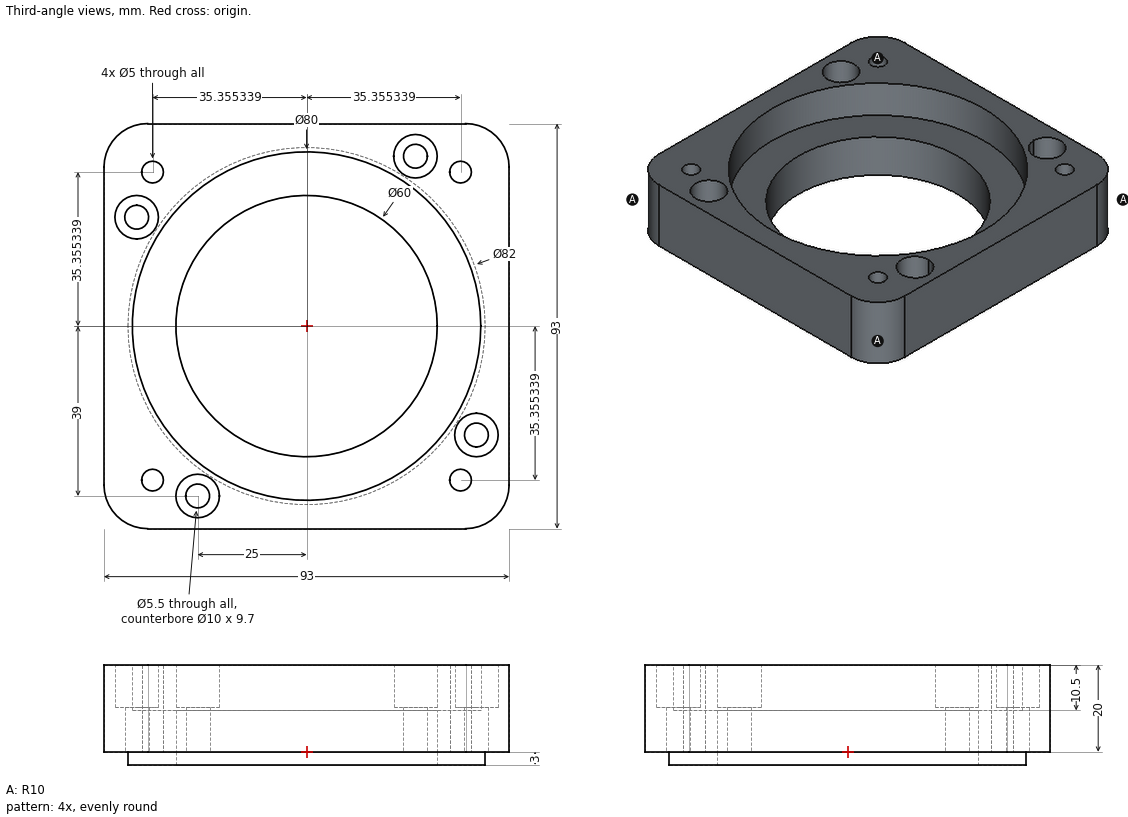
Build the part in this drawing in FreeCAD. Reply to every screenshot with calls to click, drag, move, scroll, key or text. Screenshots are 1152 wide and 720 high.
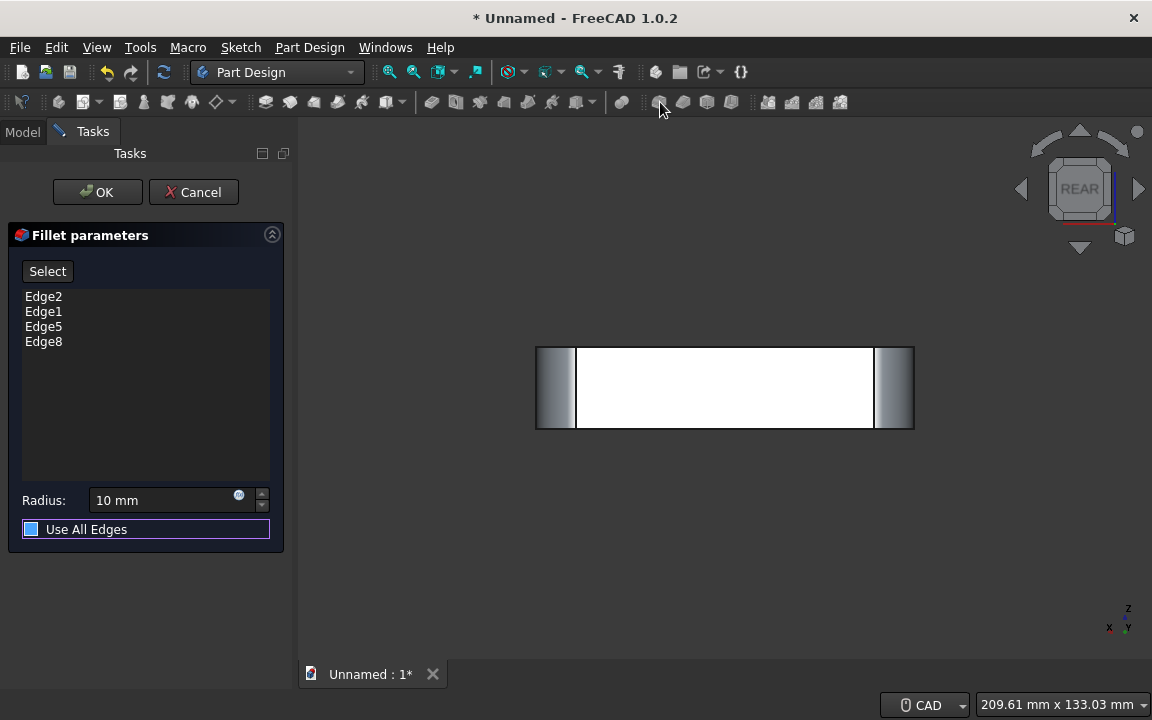
click(98, 192)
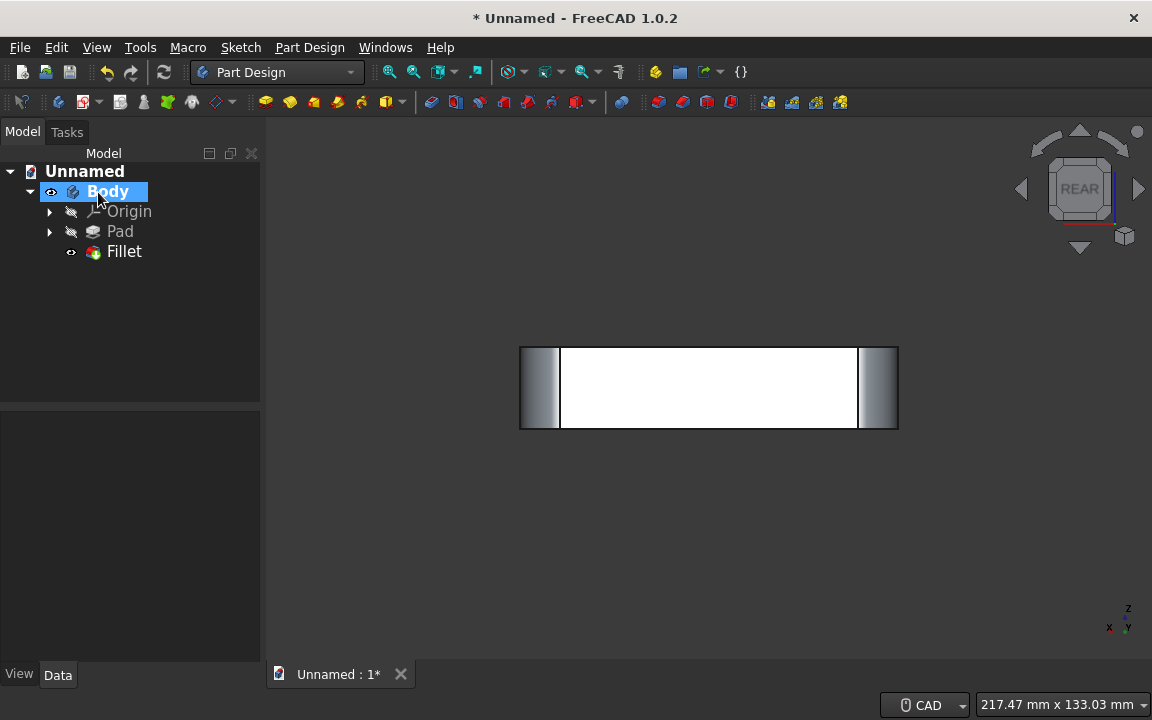
click(390, 72)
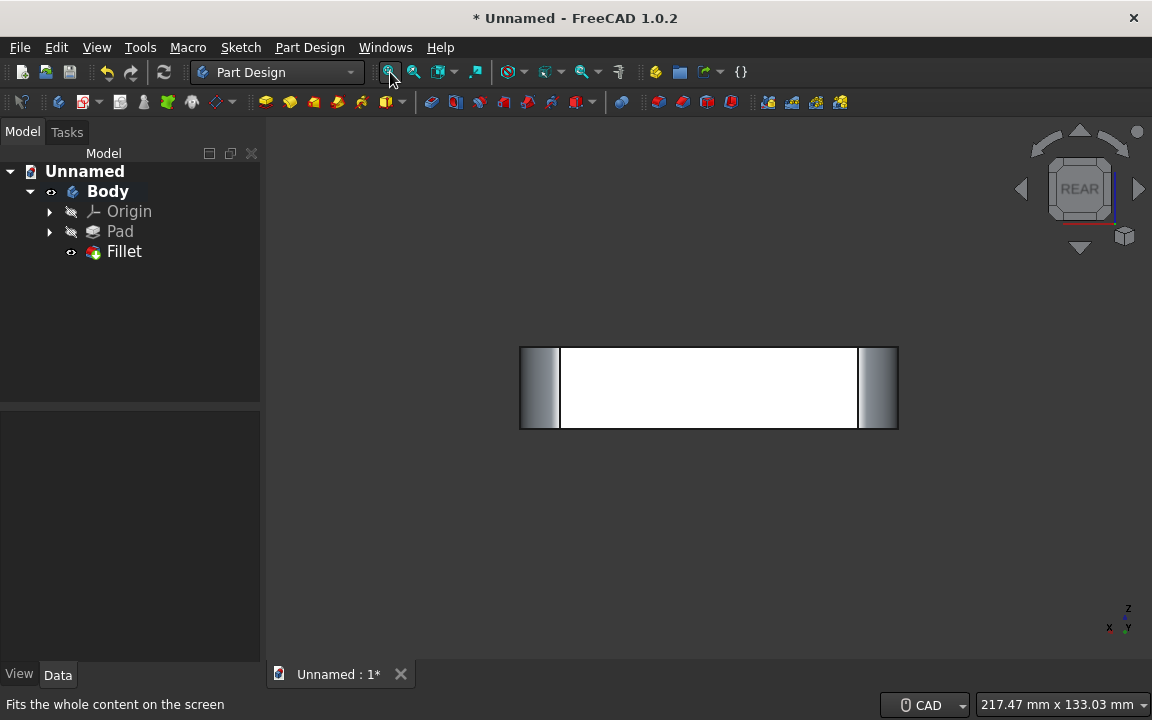
click(50, 212)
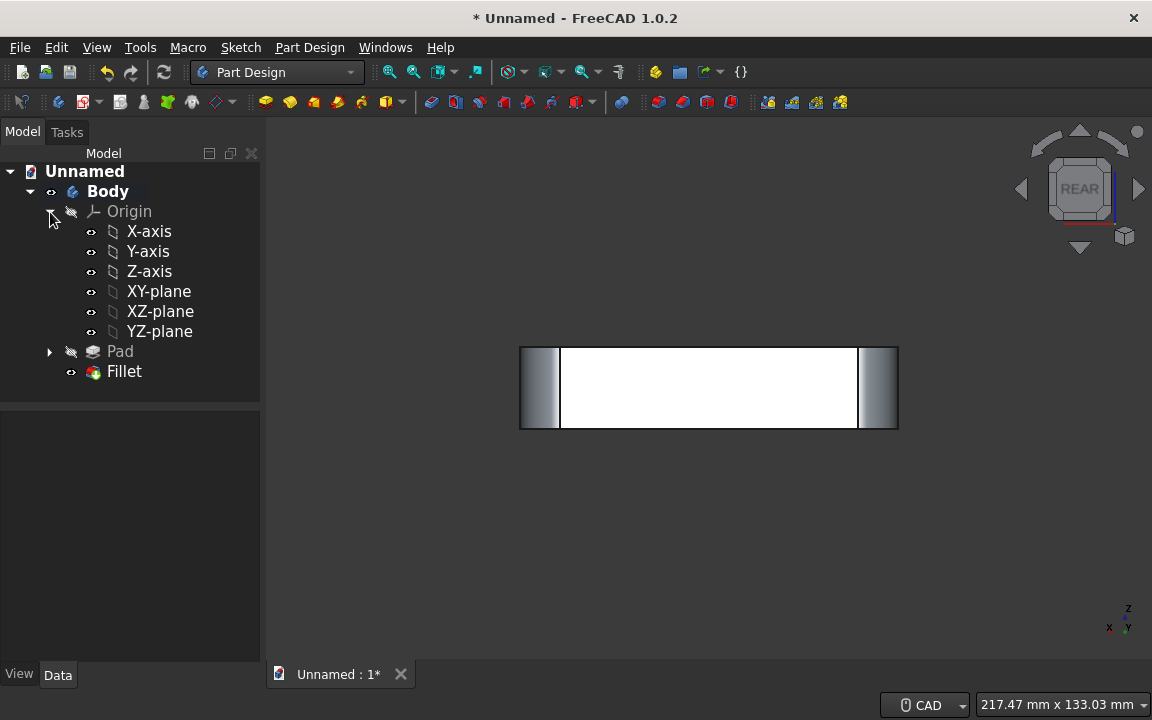
click(136, 292)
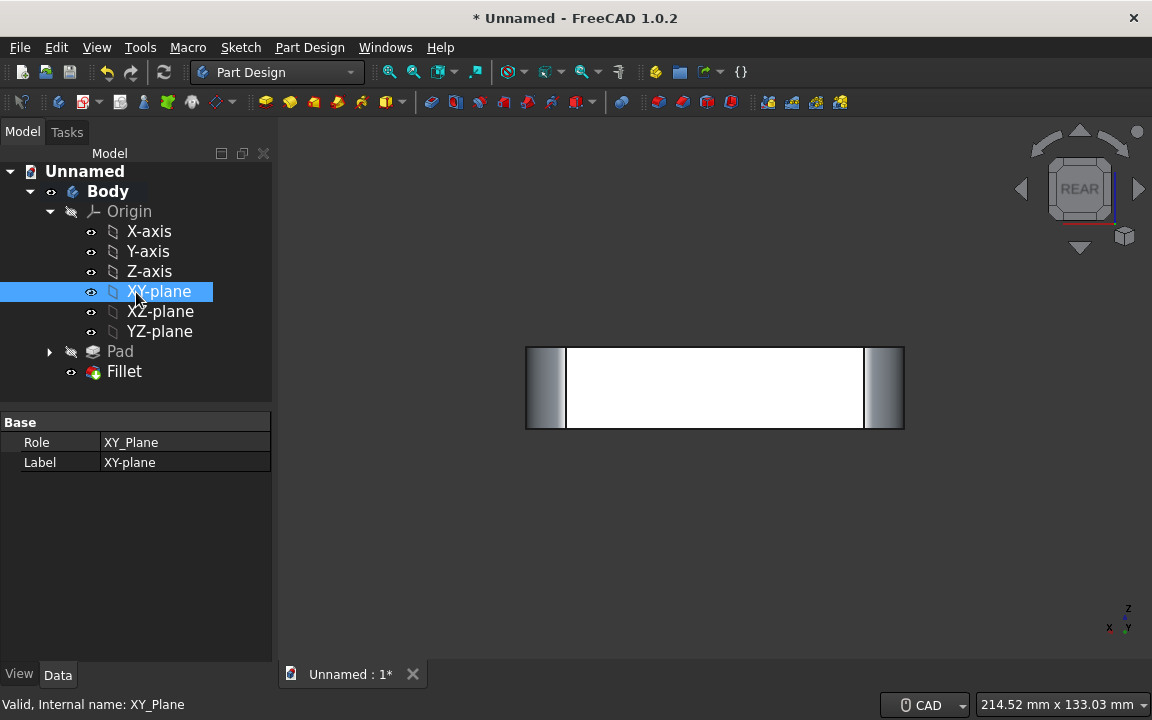
click(216, 102)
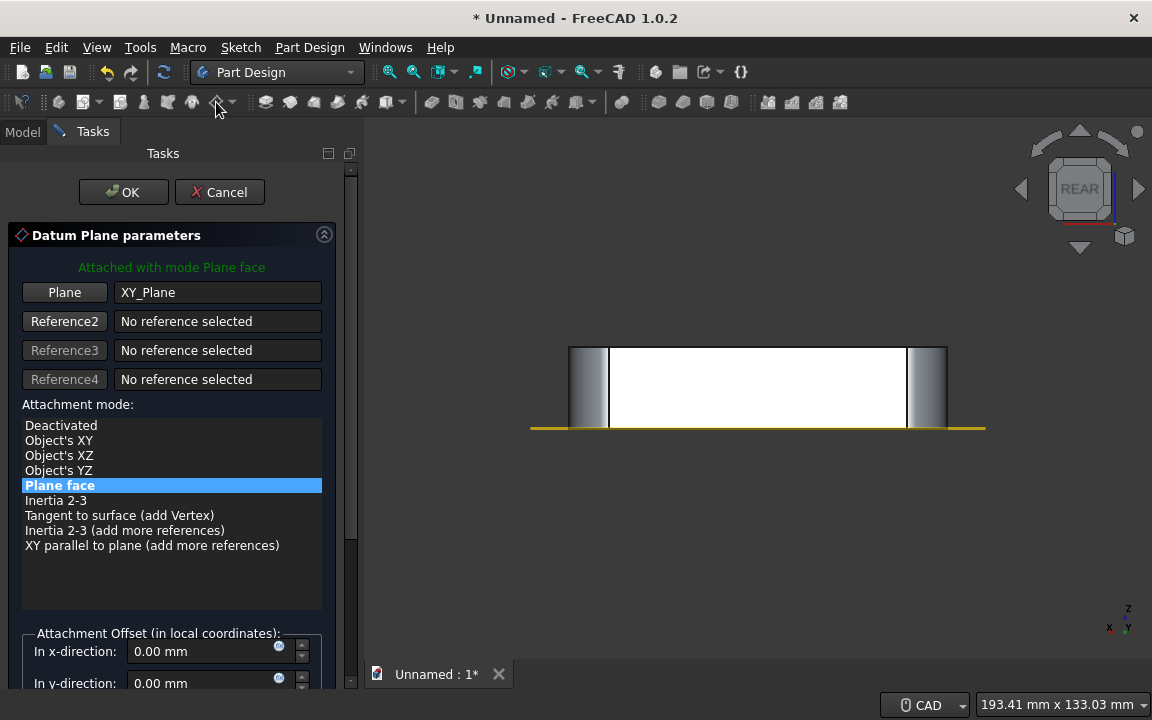
scroll(351, 426, down, 2)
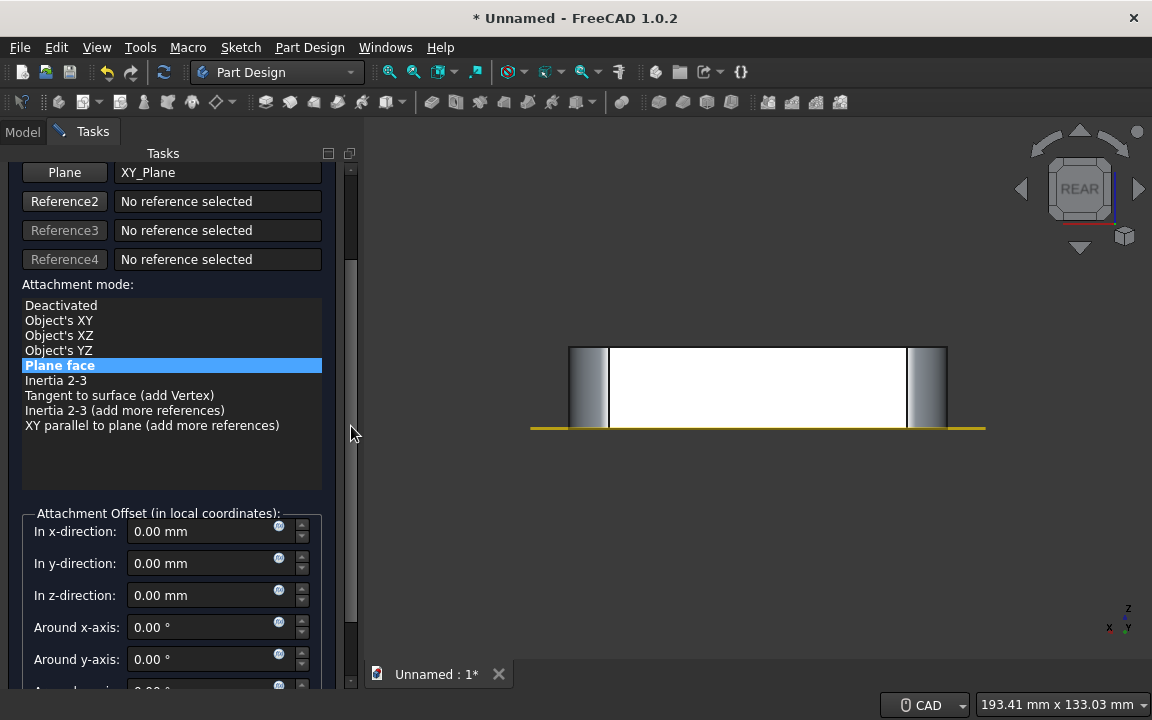
triple_click(210, 595)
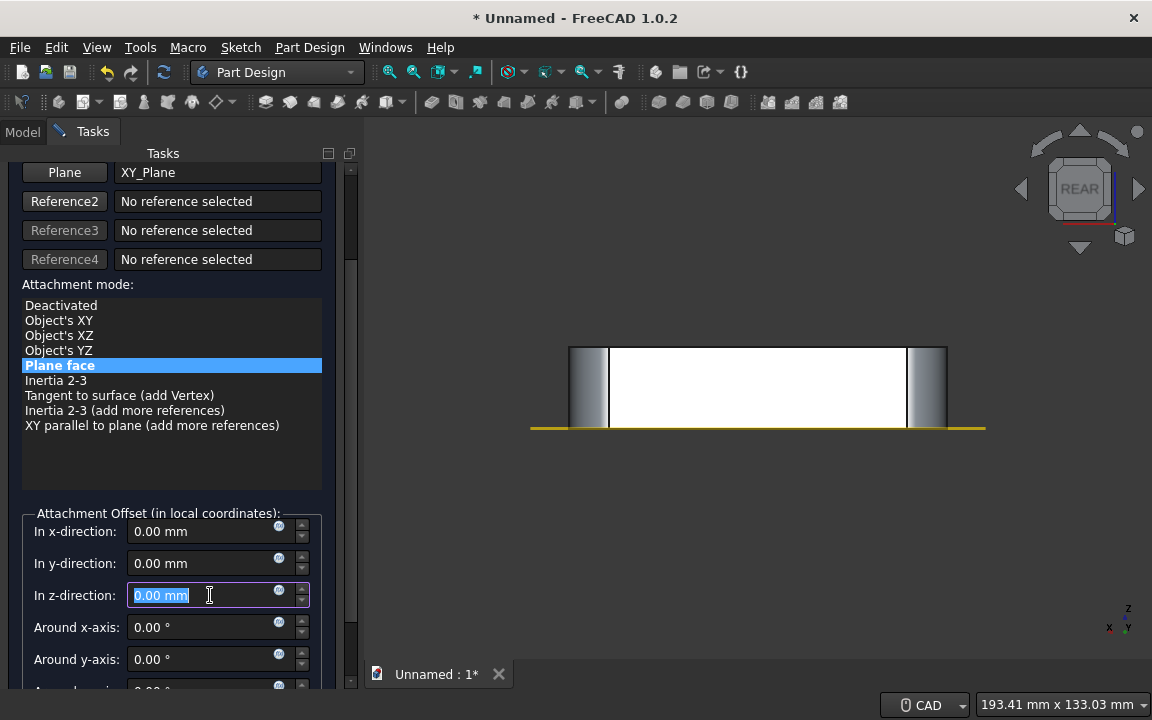
text(-3)
key(Tab)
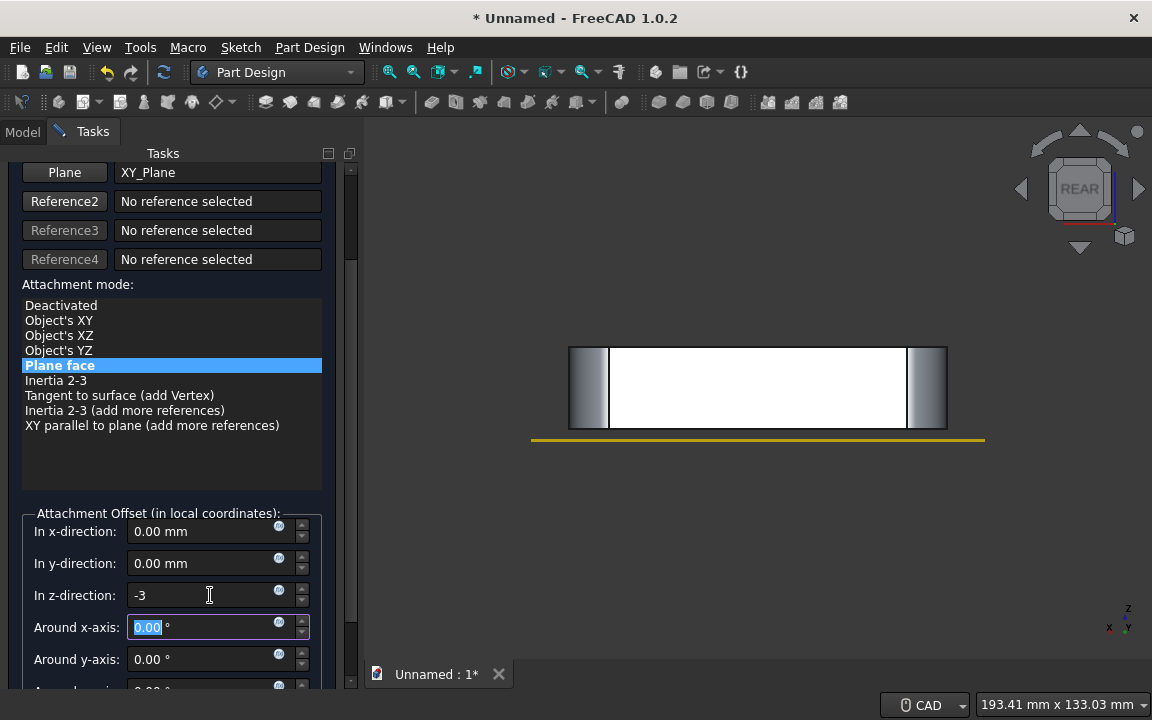
scroll(351, 426, up, 3)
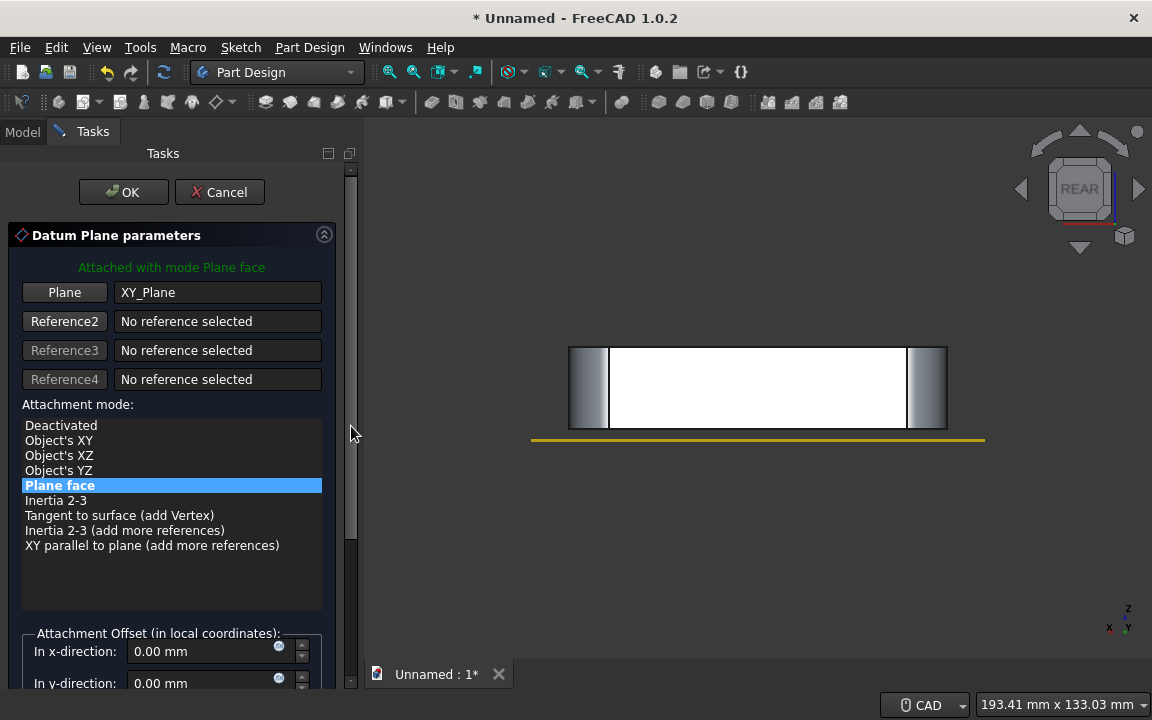
click(124, 192)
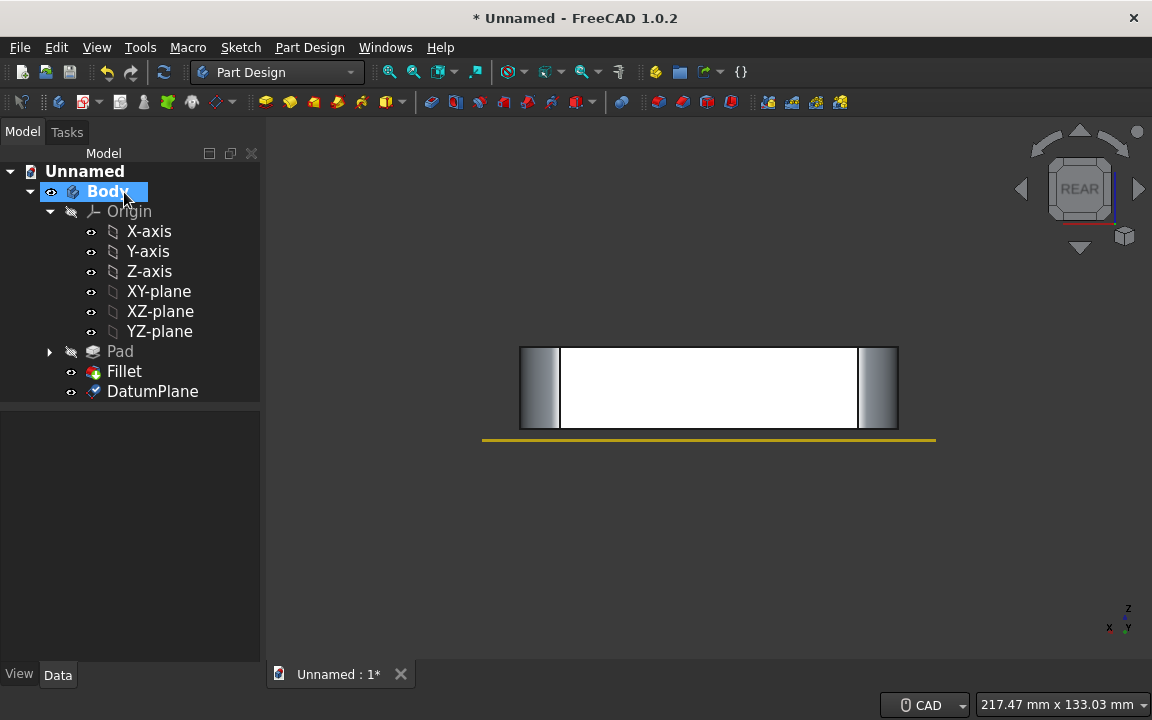
click(116, 392)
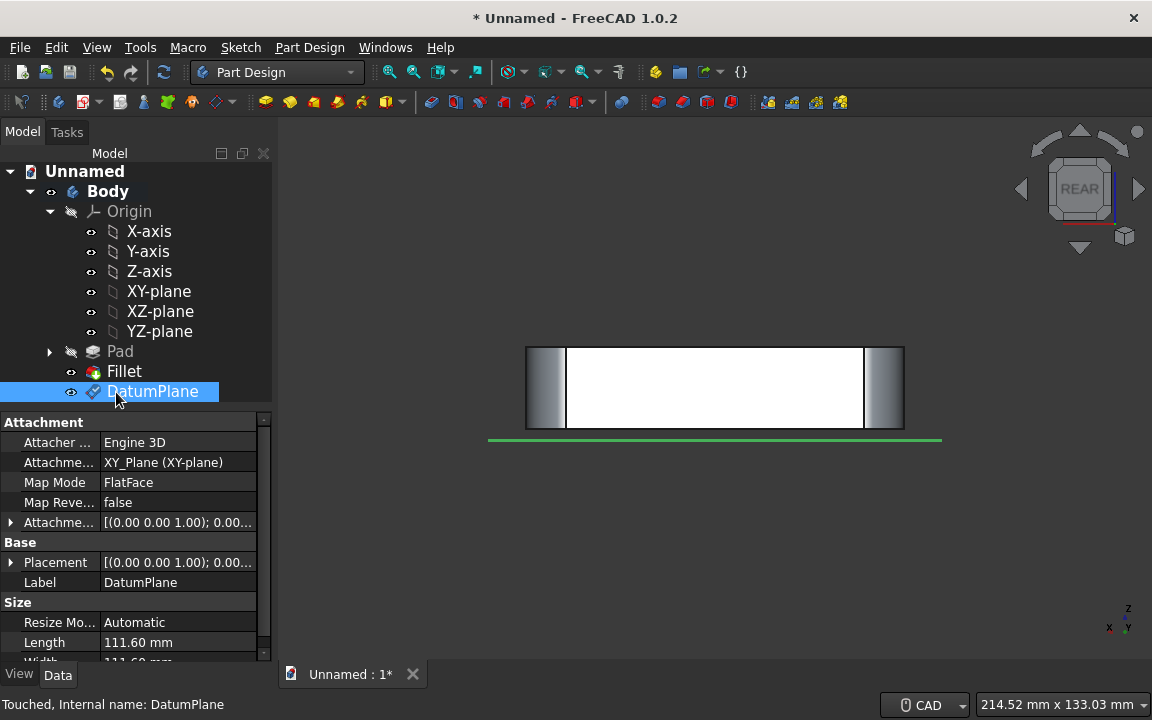
click(84, 102)